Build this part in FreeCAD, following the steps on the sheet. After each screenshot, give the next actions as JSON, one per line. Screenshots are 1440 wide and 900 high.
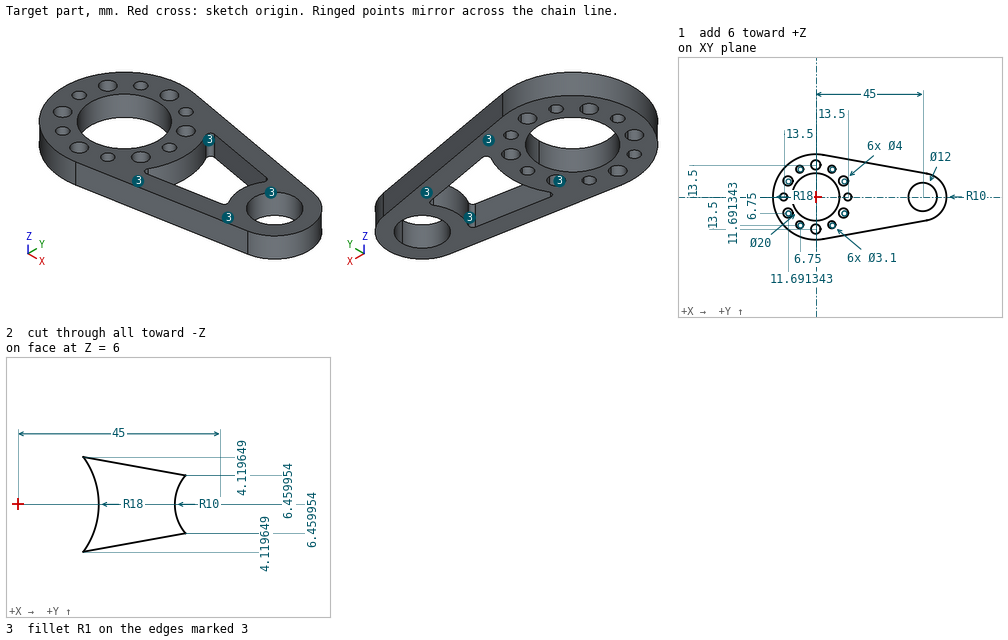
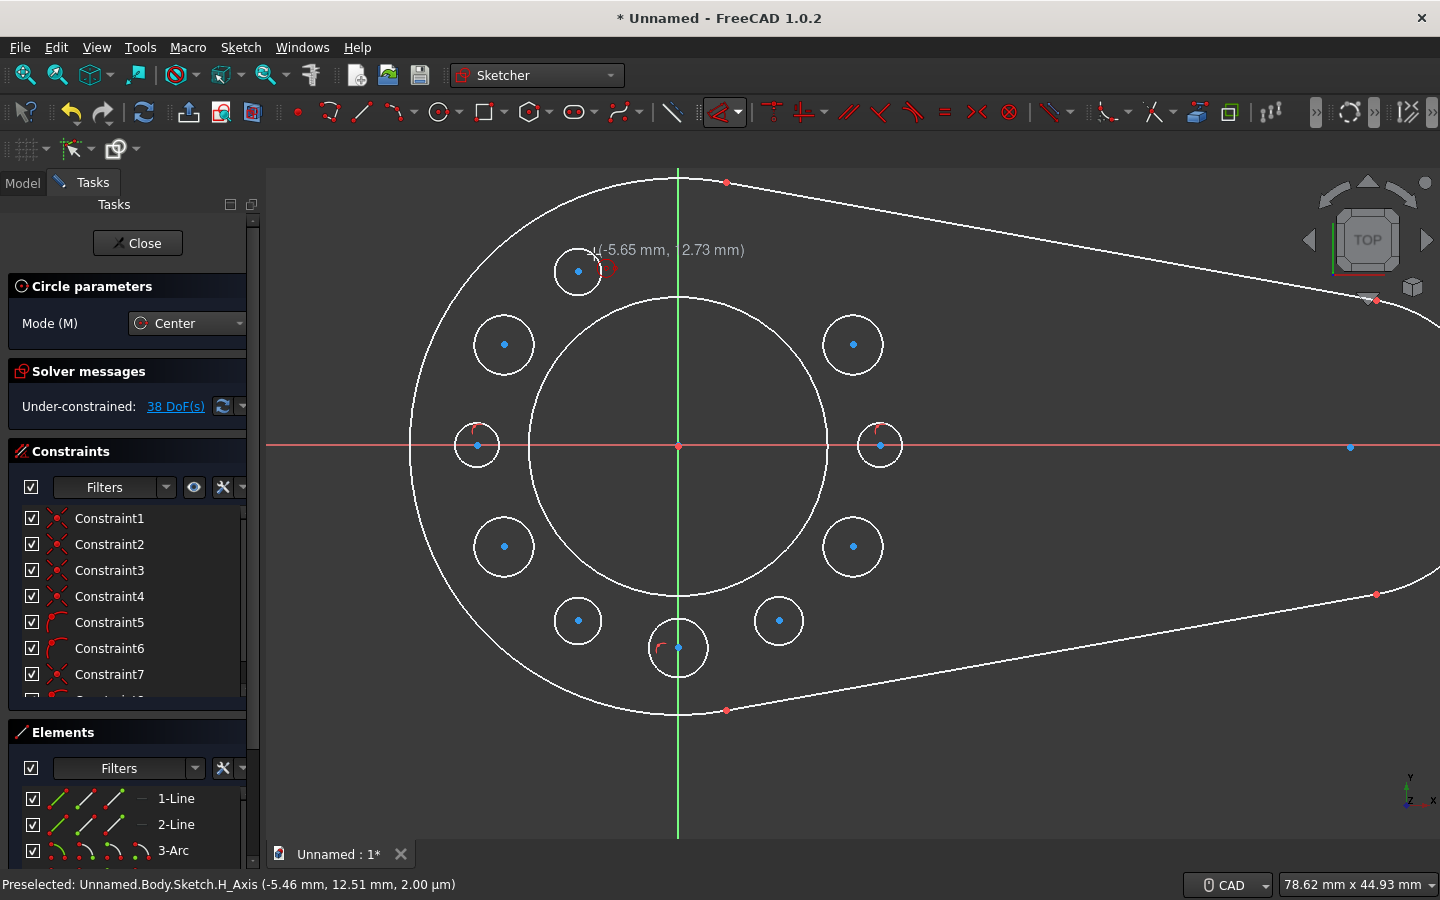
{"action": "left_click", "coordinate": [678, 244]}
{"action": "left_click", "coordinate": [699, 222]}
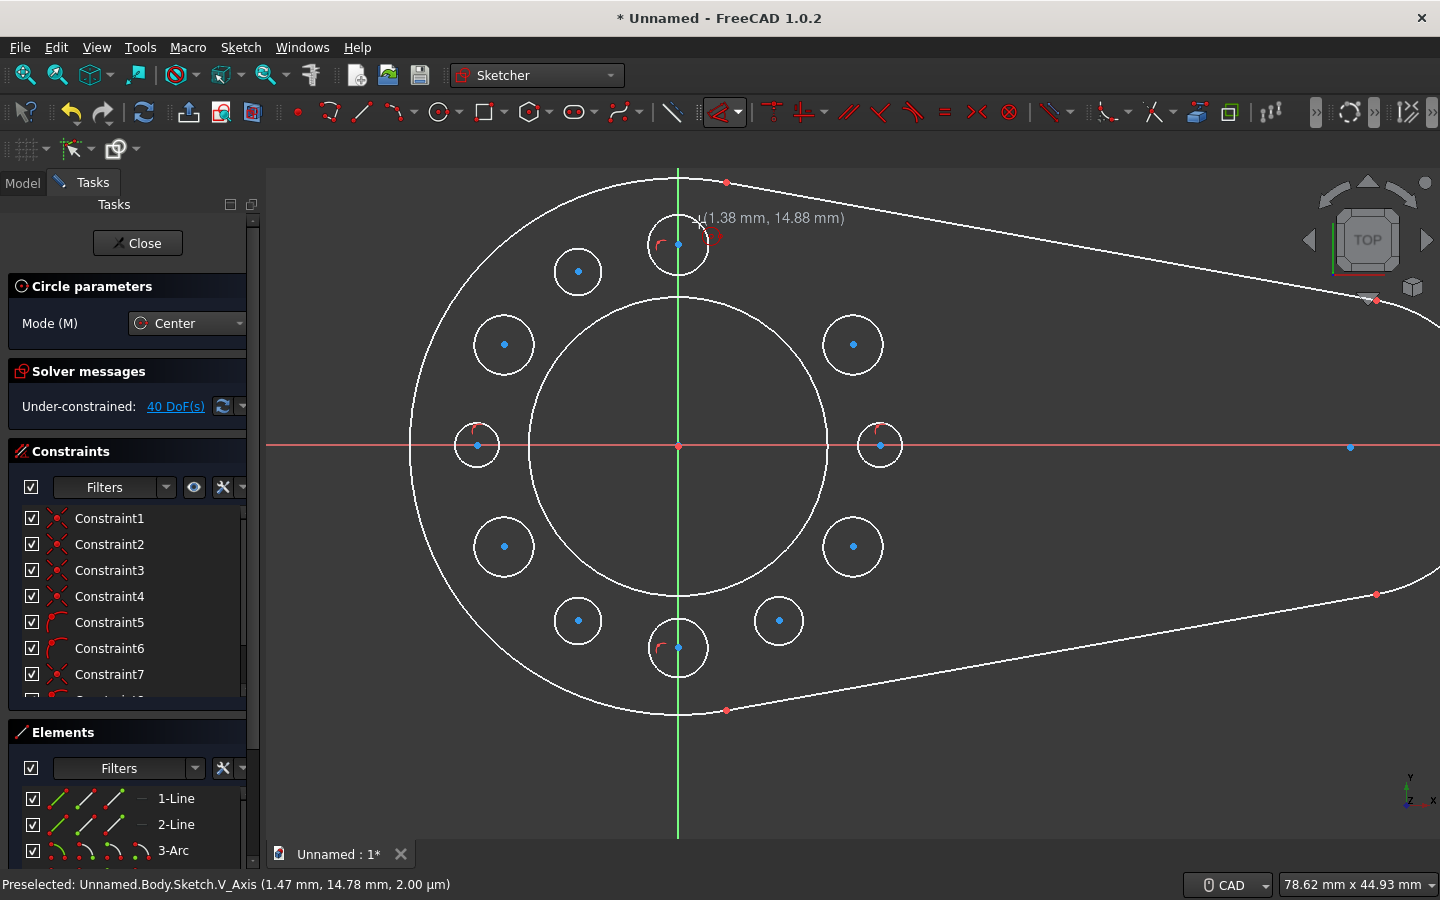
{"action": "left_click", "coordinate": [779, 271]}
{"action": "left_click", "coordinate": [796, 254]}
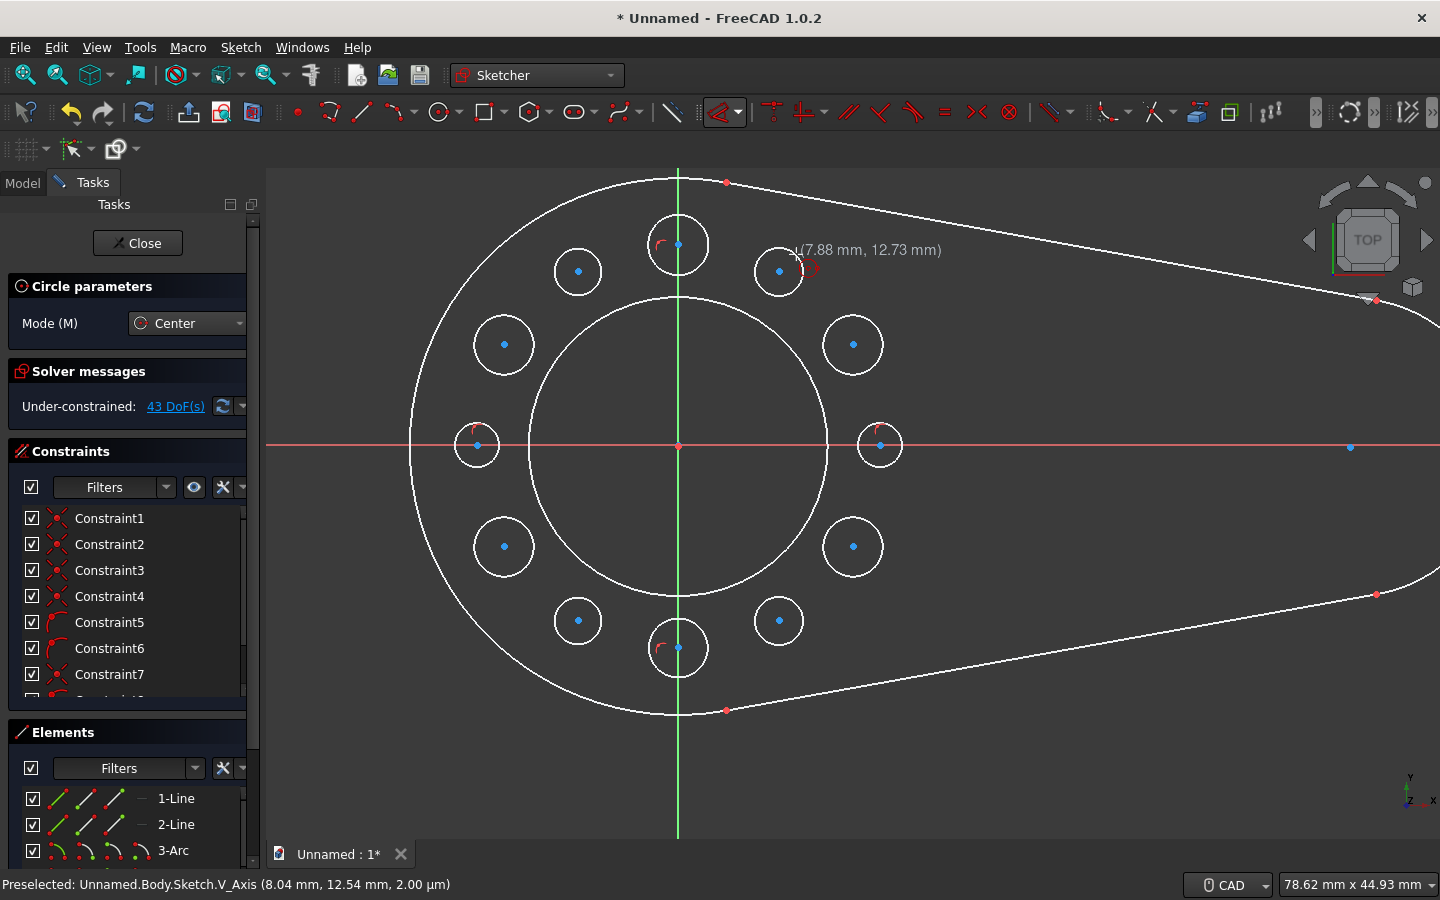
{"action": "scroll", "coordinate": [439, 622], "scroll_direction": "down", "scroll_amount": 2}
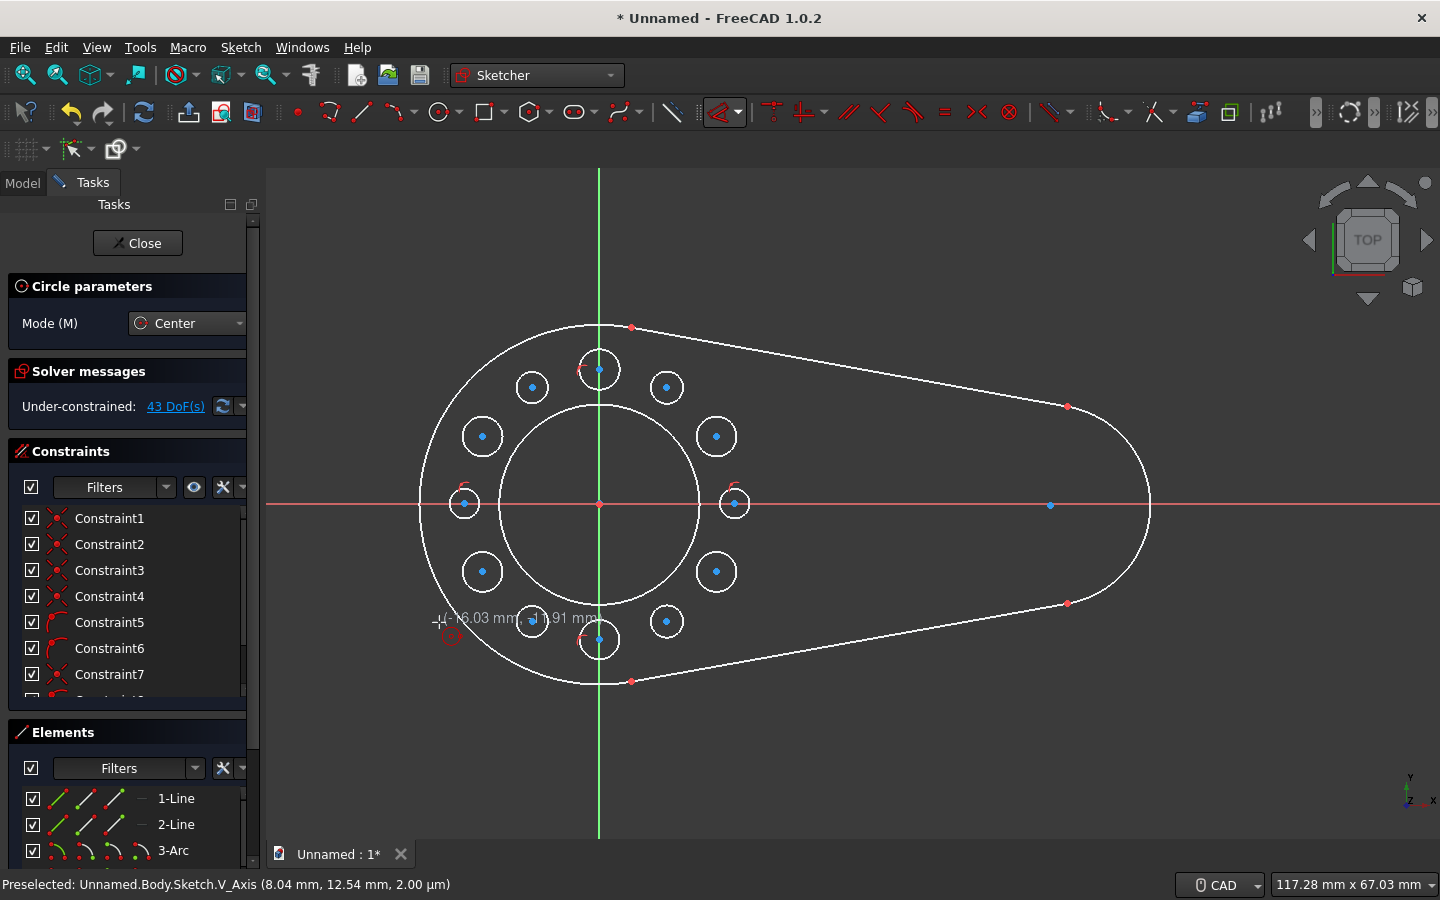
{"action": "left_click", "coordinate": [1050, 504]}
{"action": "left_click", "coordinate": [1092, 461]}
{"action": "key", "text": "Escape"}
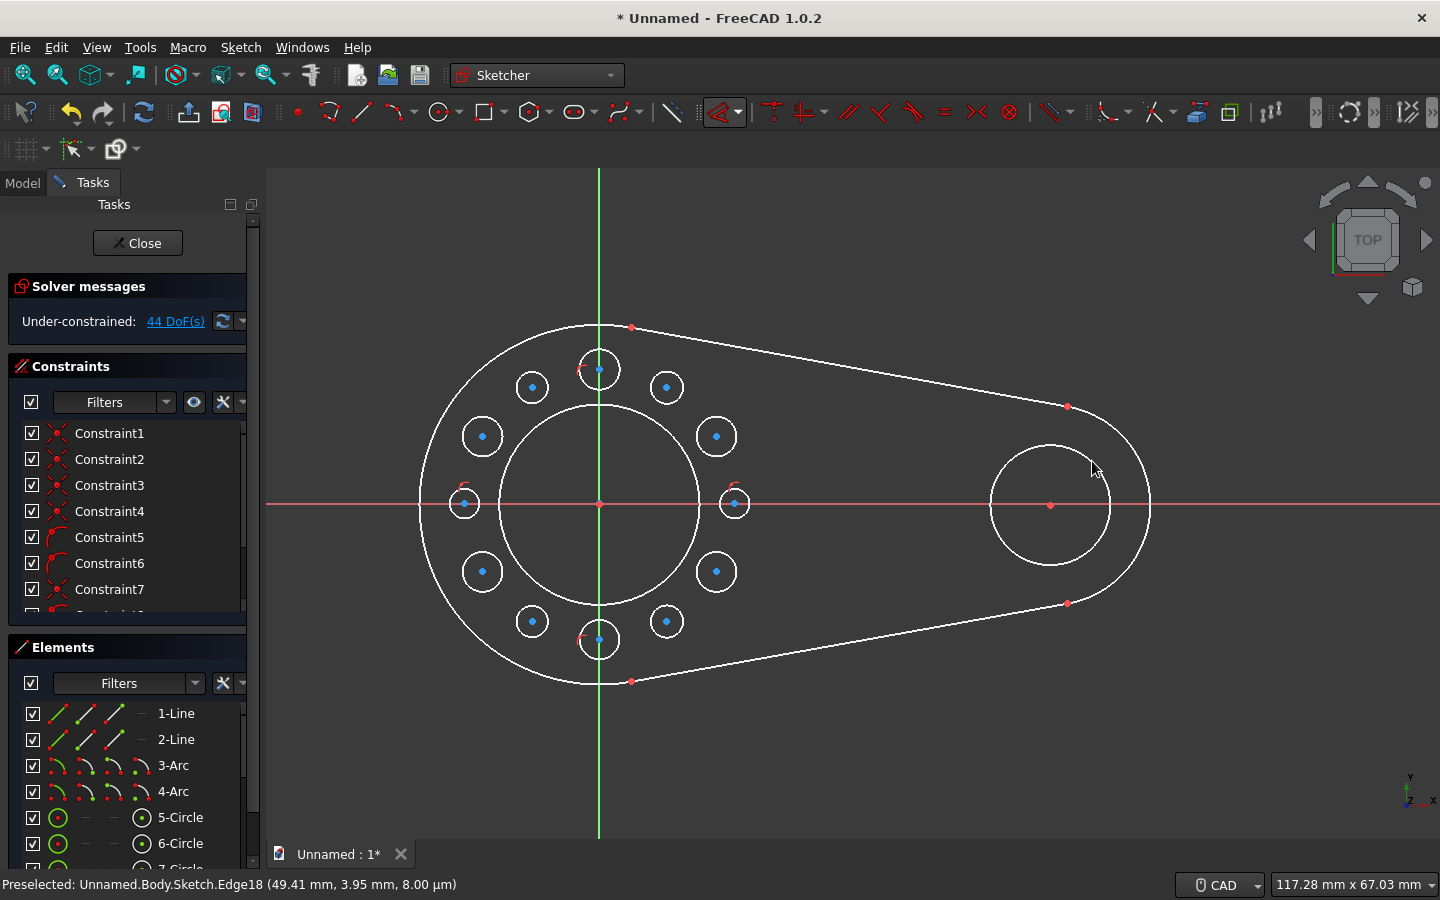
{"action": "left_click", "coordinate": [937, 383]}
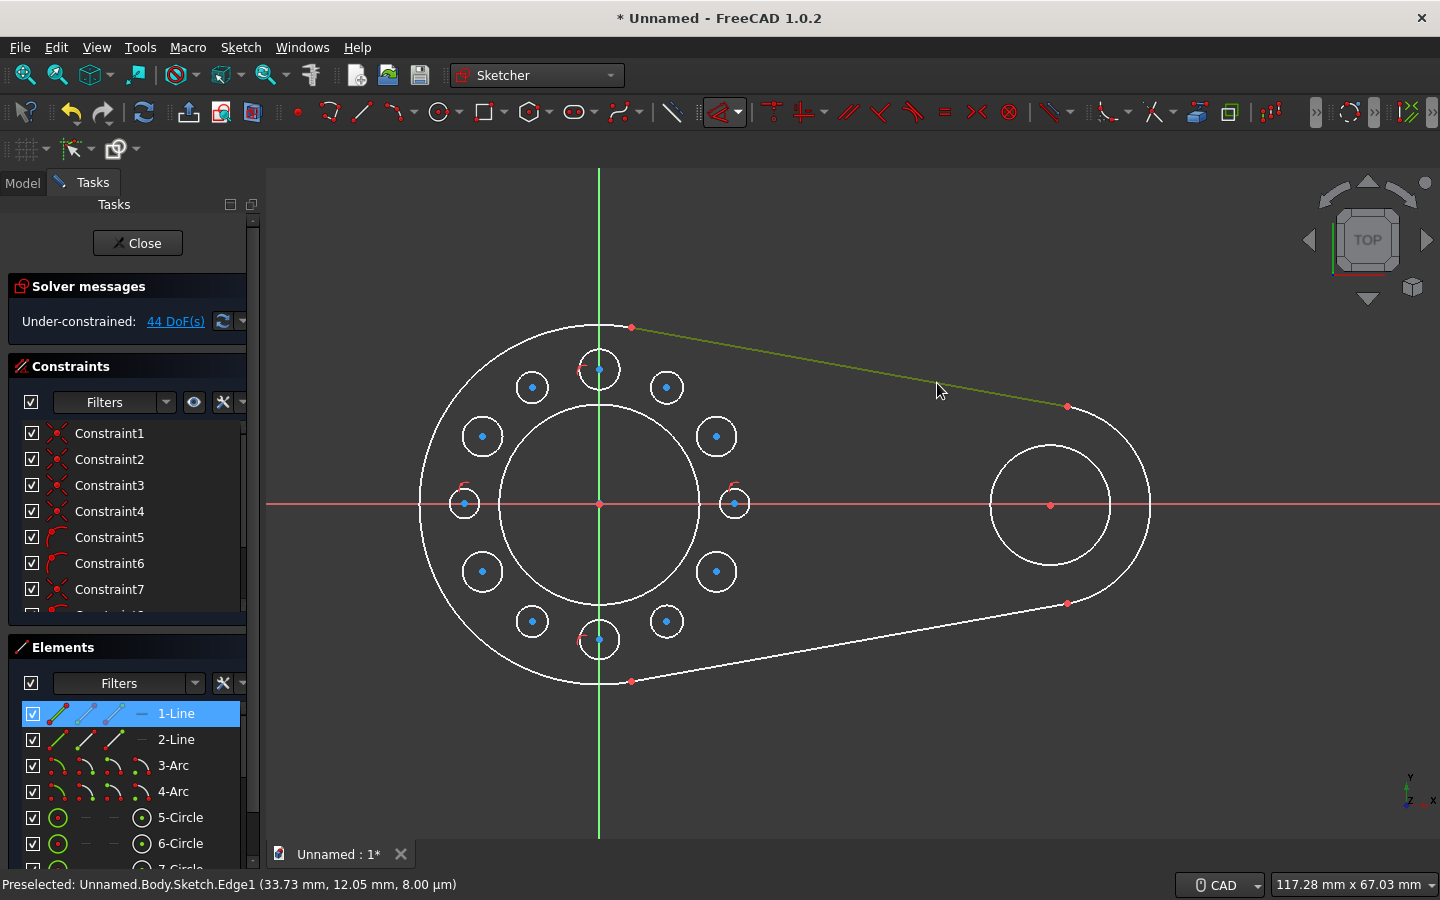
{"action": "left_click", "coordinate": [462, 389]}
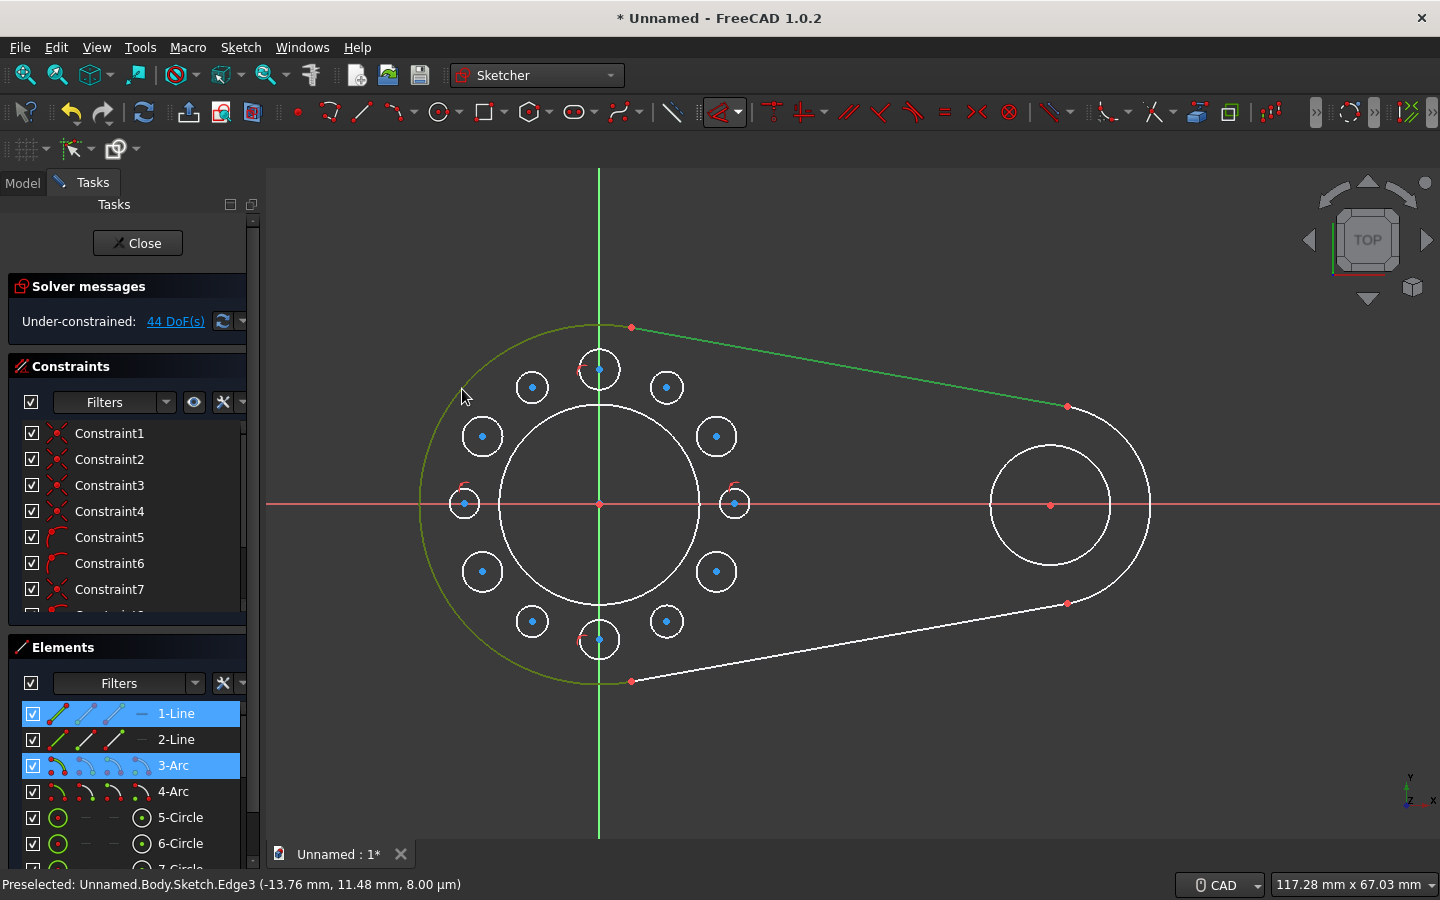
{"action": "key", "text": "t"}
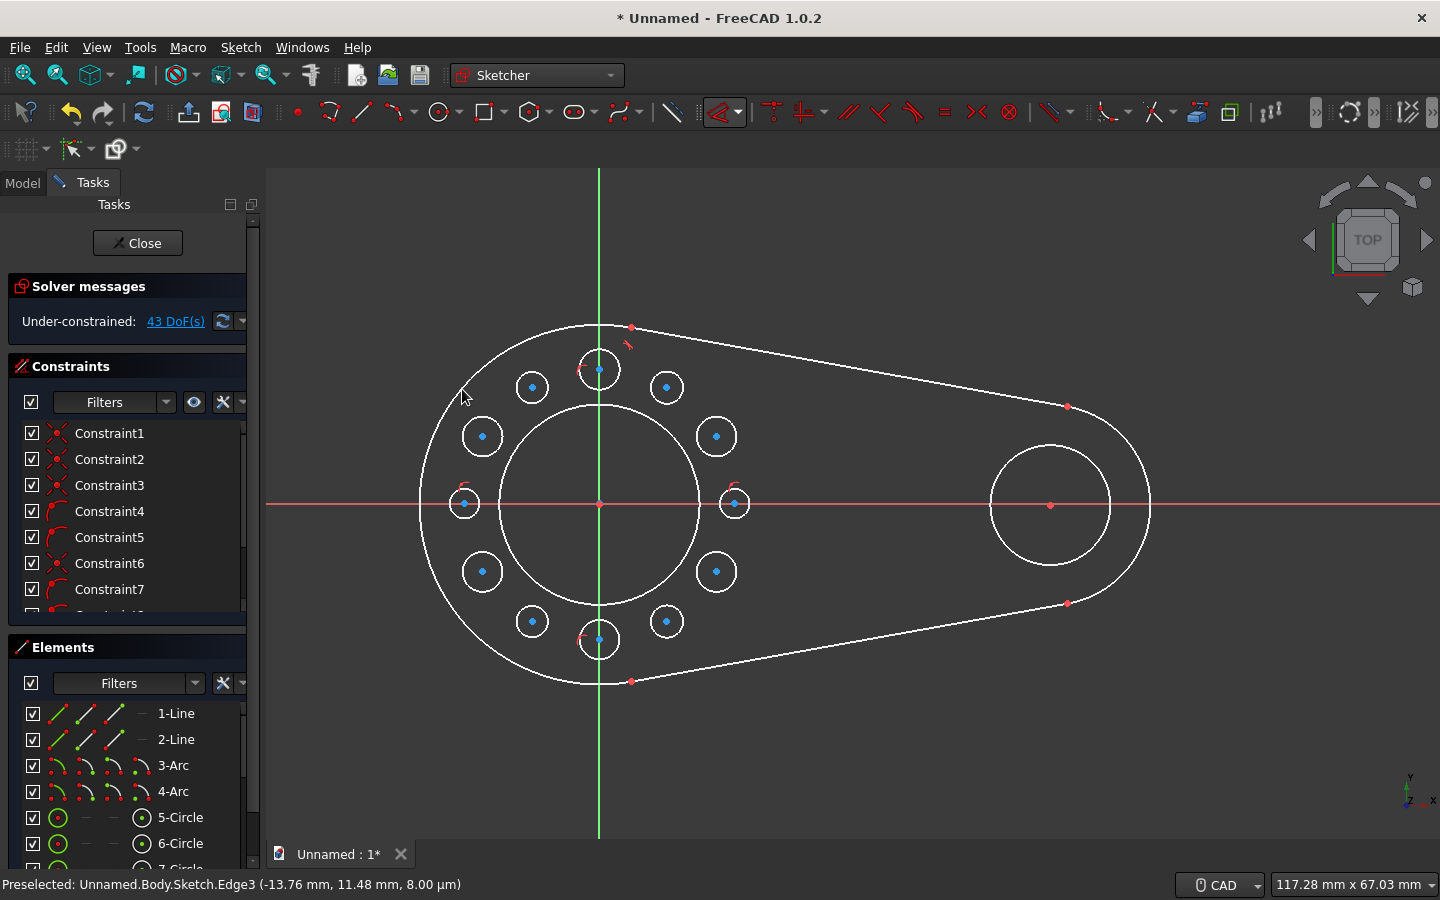
{"action": "left_click", "coordinate": [937, 383]}